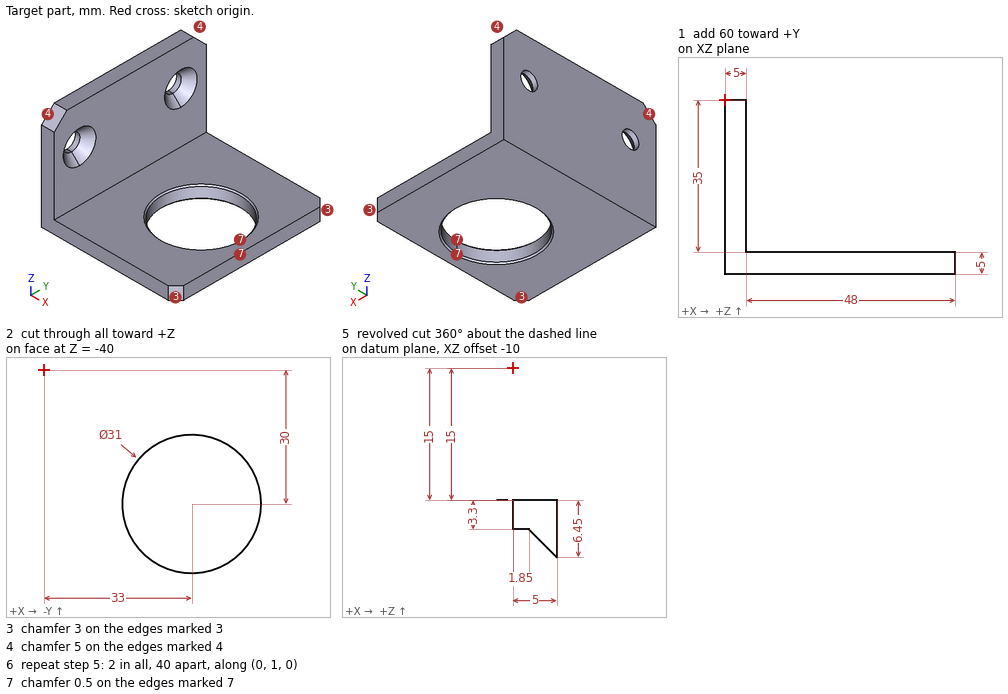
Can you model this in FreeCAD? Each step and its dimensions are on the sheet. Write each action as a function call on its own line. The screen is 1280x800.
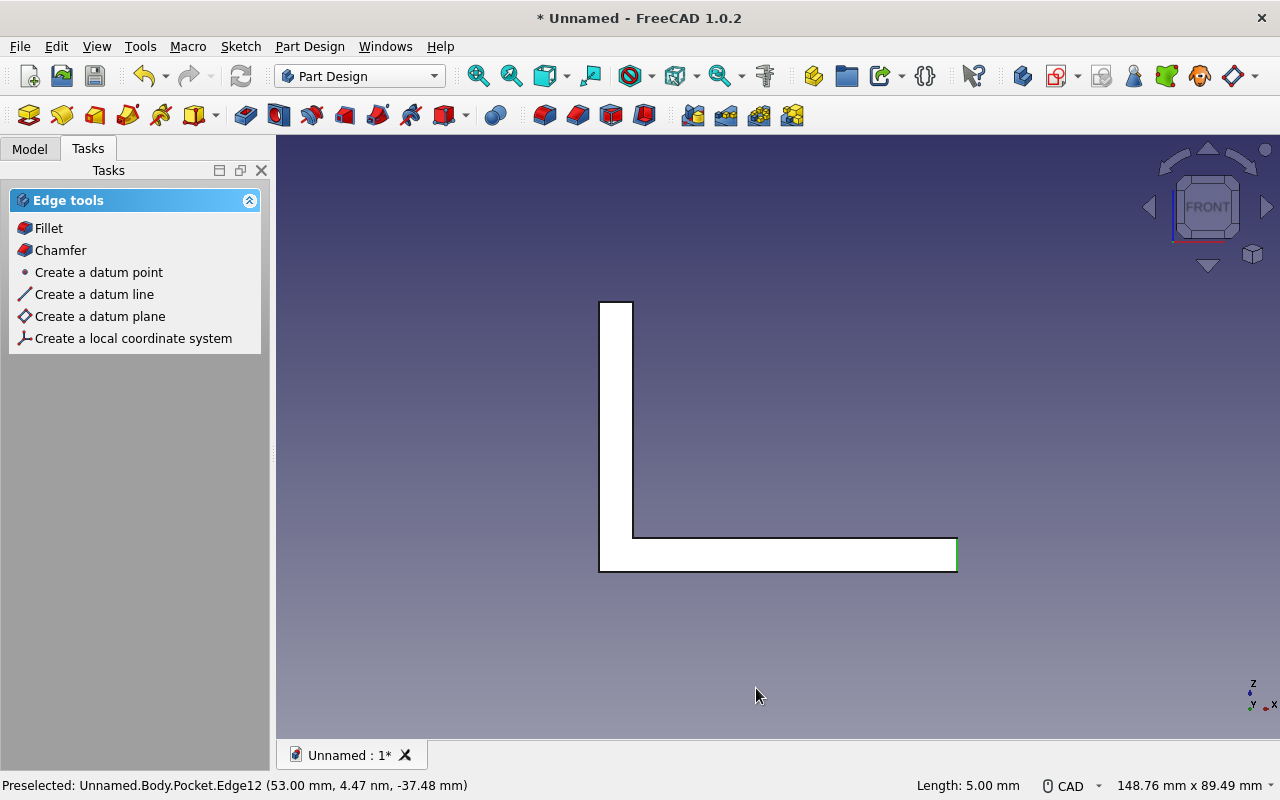
key(v)
key(f)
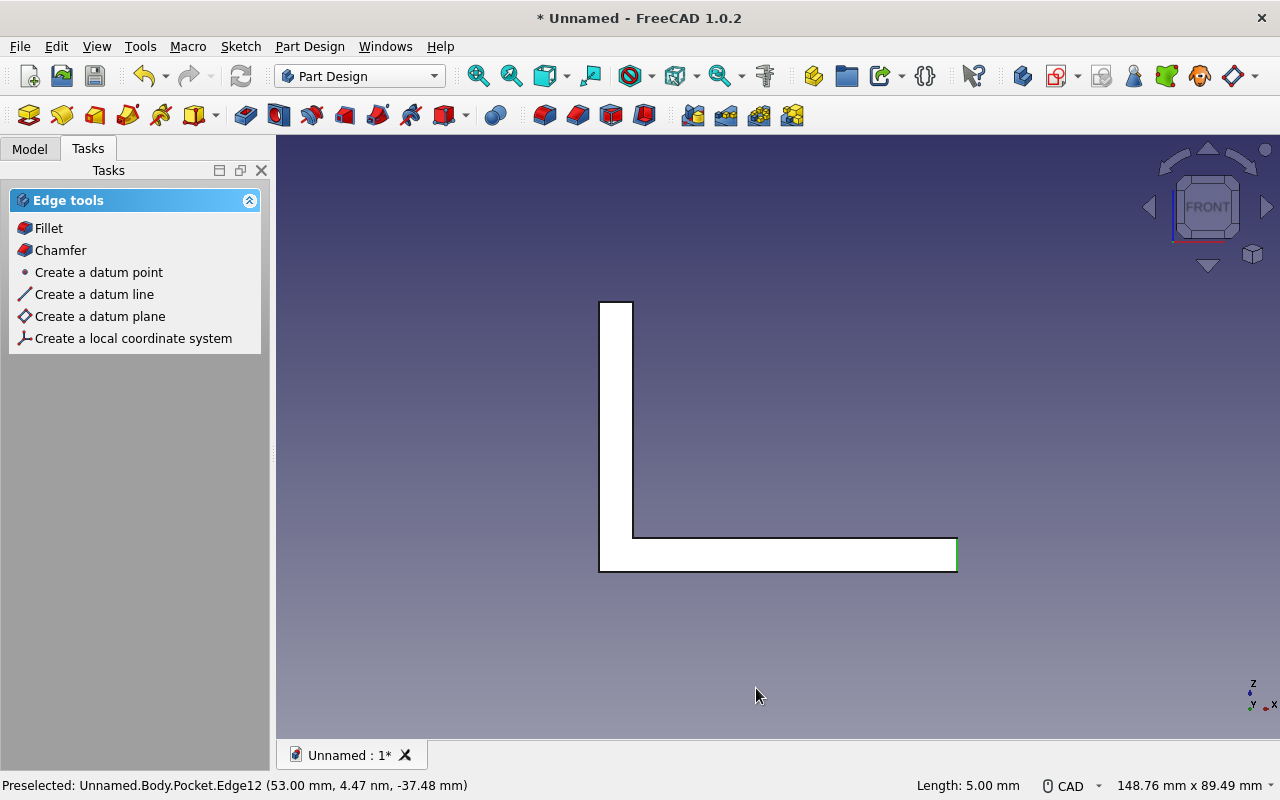
key(3)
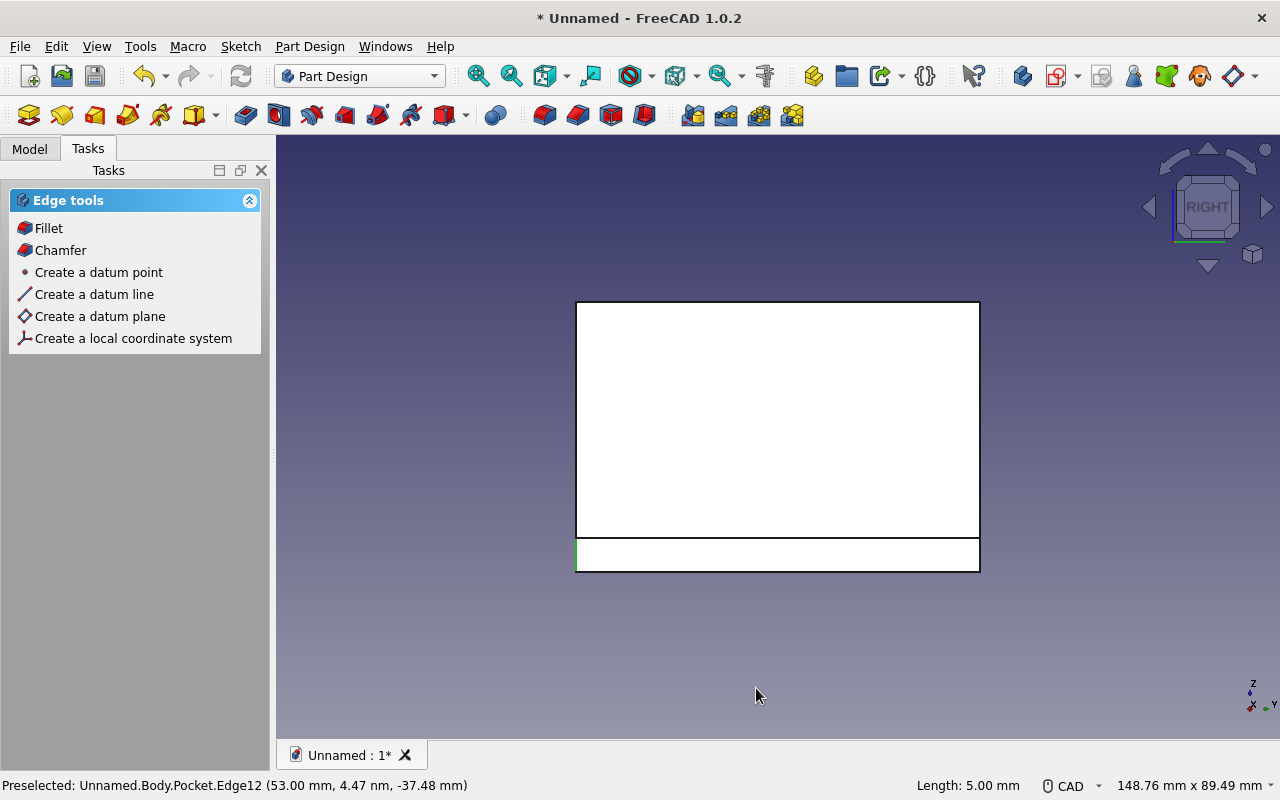
key(v)
key(f)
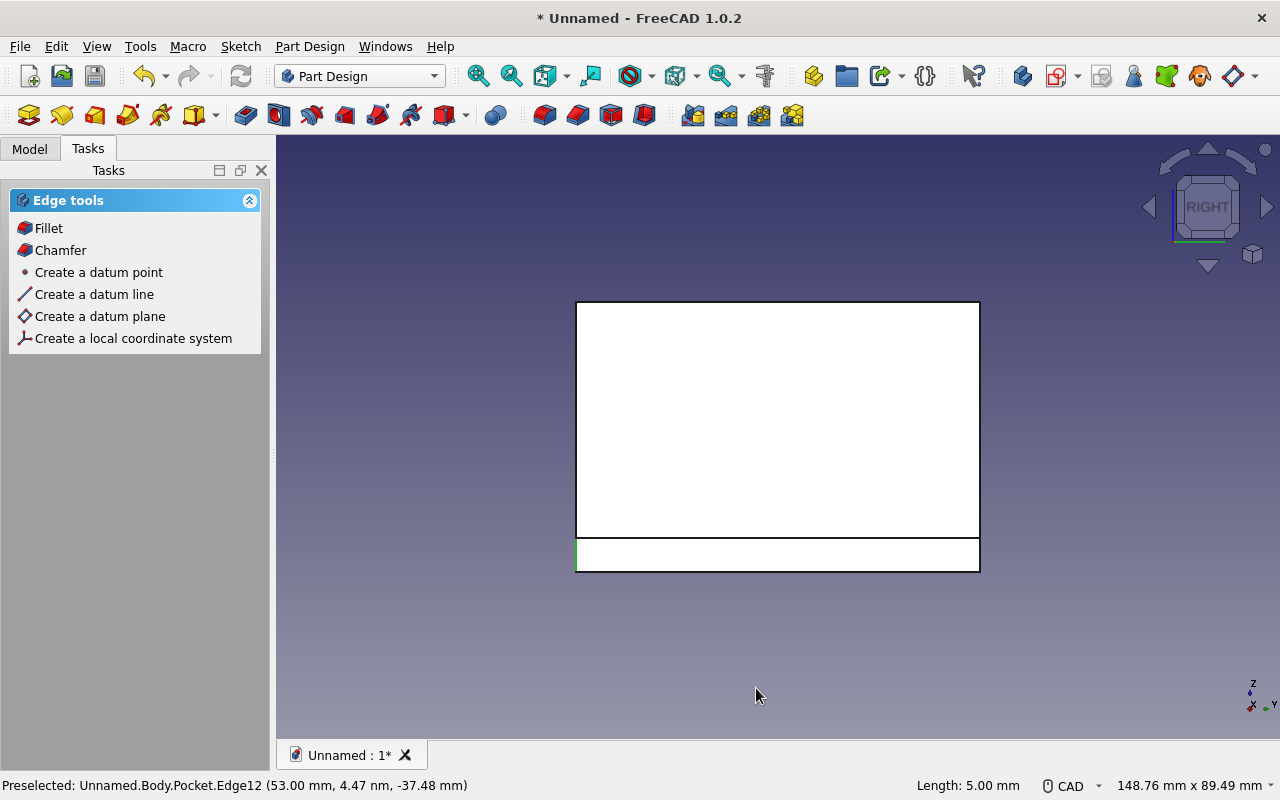
click(980, 554, ctrl)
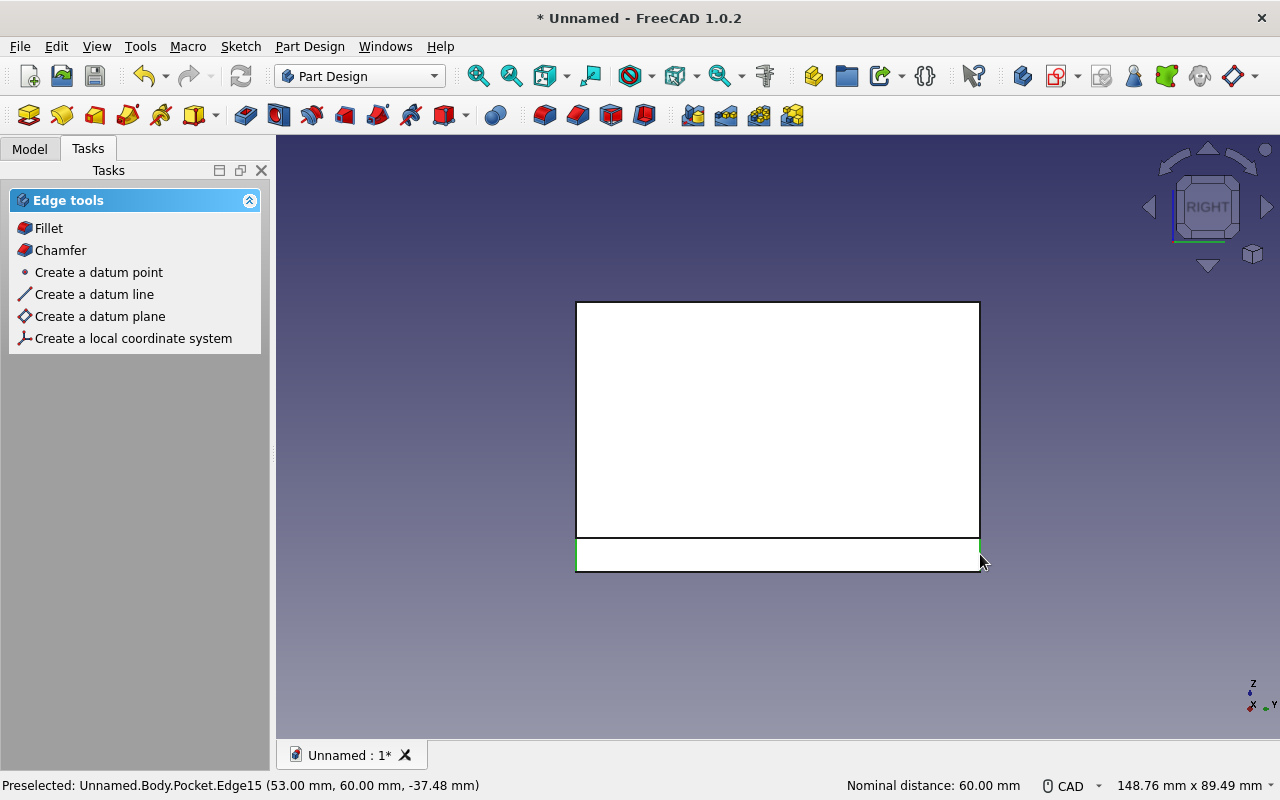
click(578, 116)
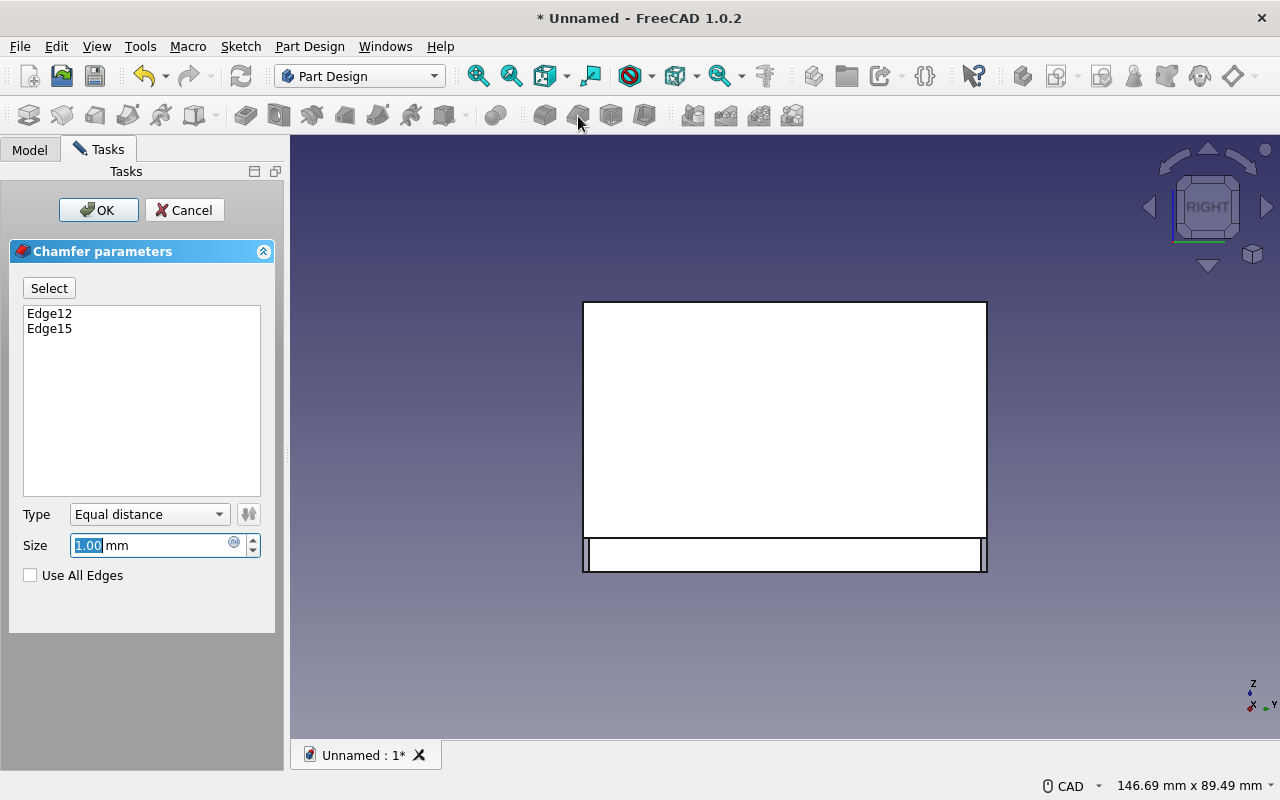
text(3)
key(Tab)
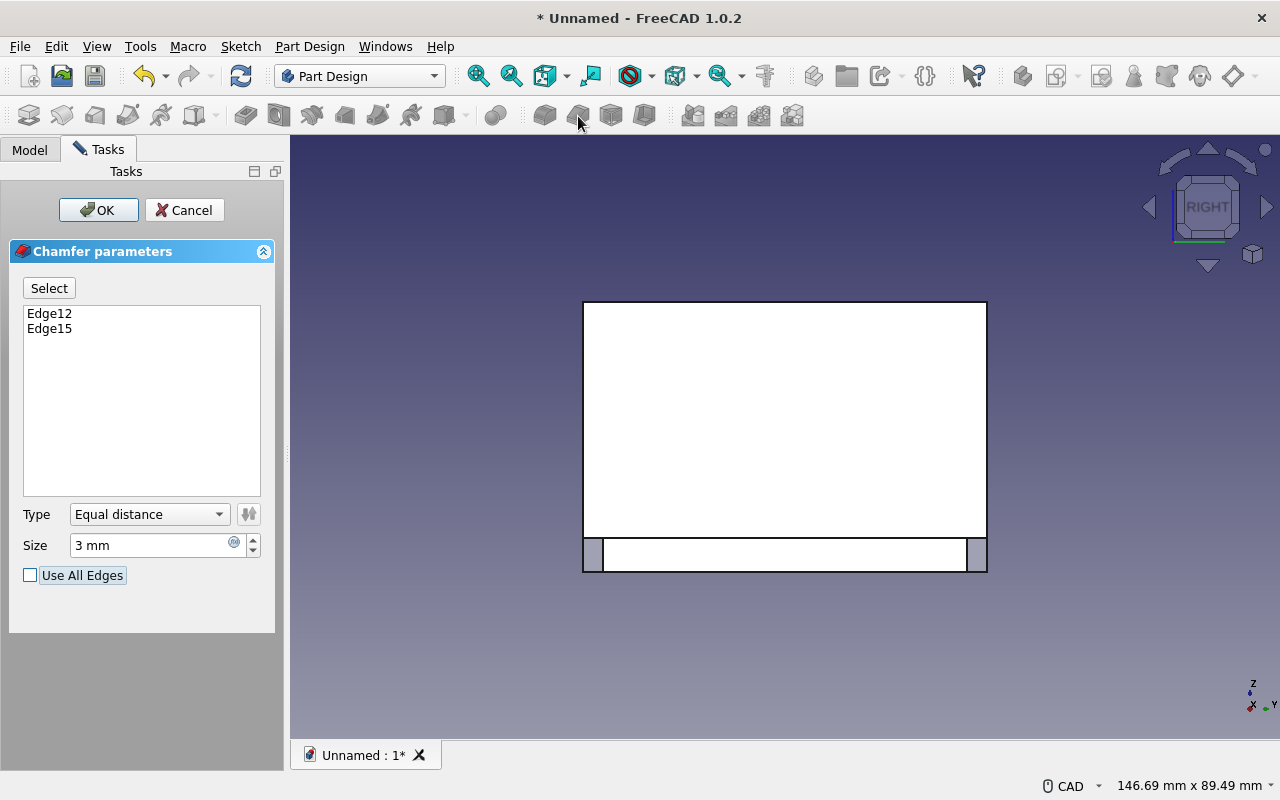
click(99, 210)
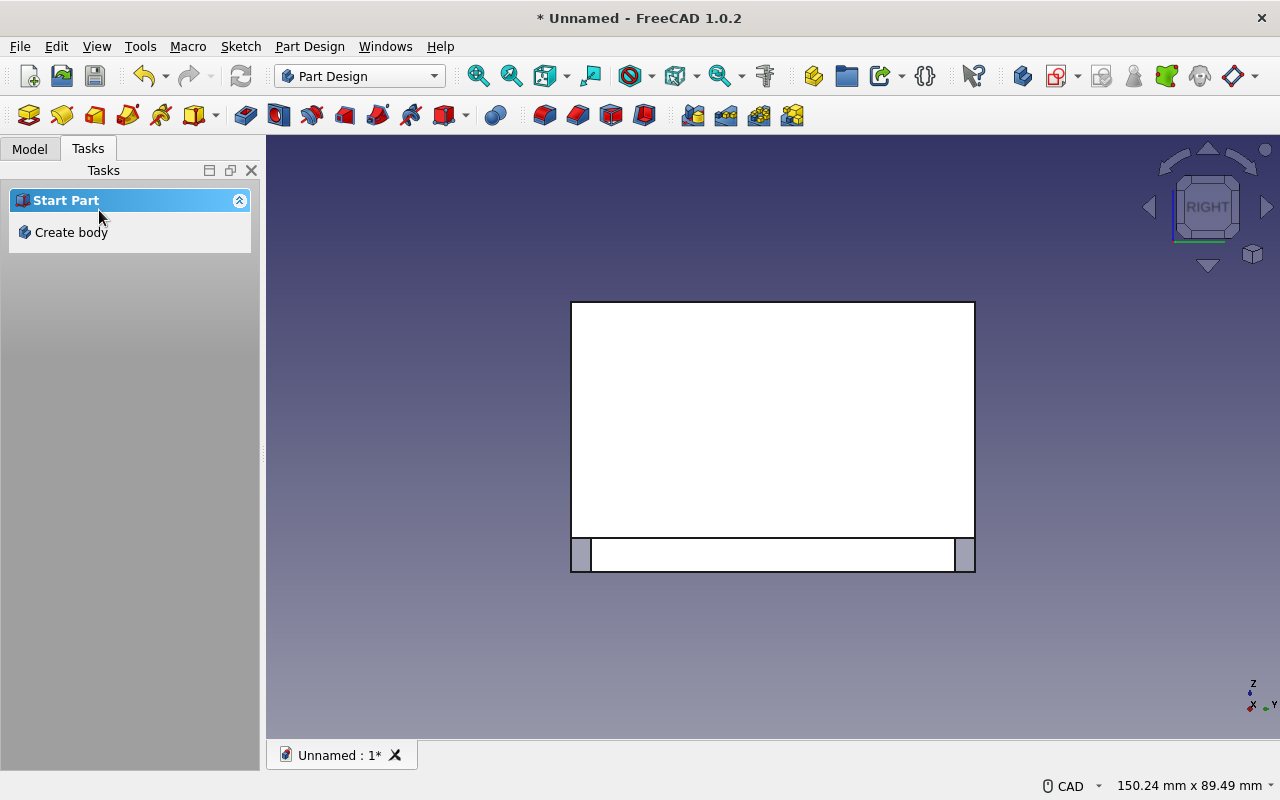
key(v)
key(f)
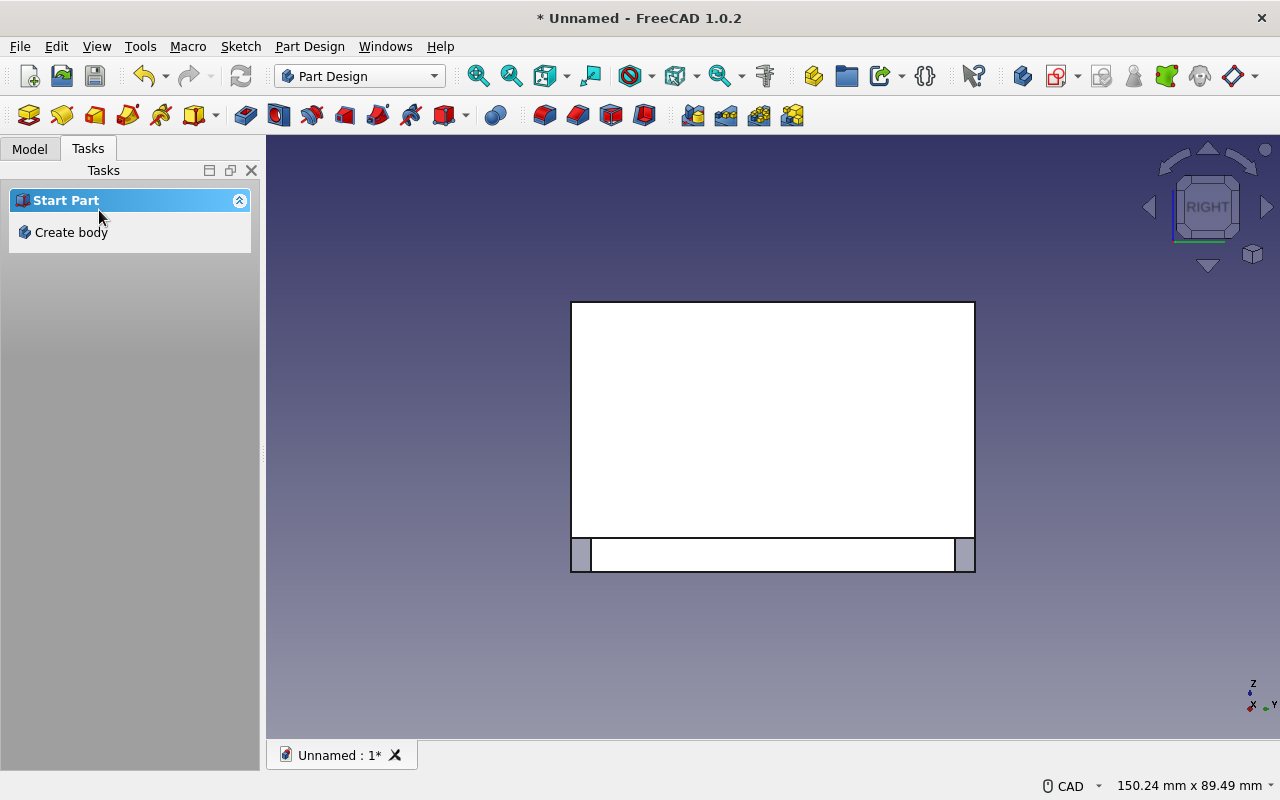
key(0)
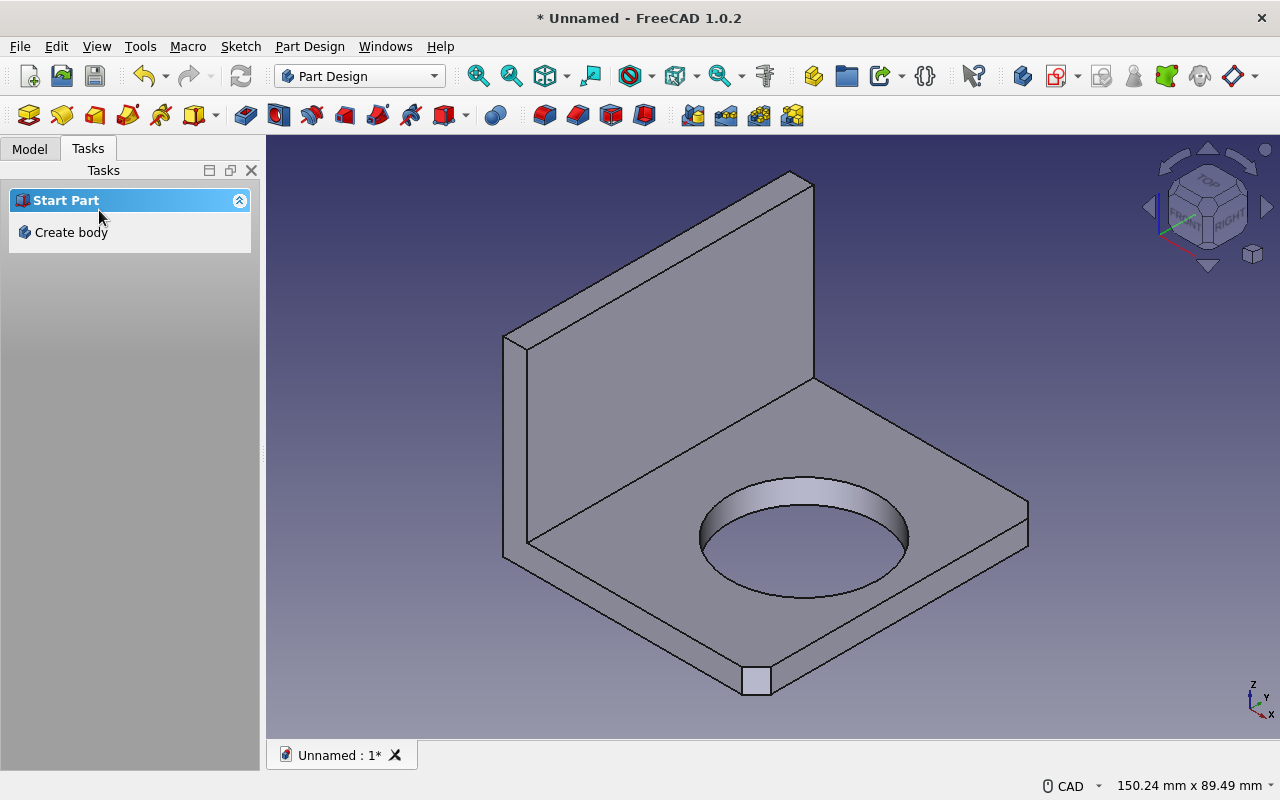
click(515, 342)